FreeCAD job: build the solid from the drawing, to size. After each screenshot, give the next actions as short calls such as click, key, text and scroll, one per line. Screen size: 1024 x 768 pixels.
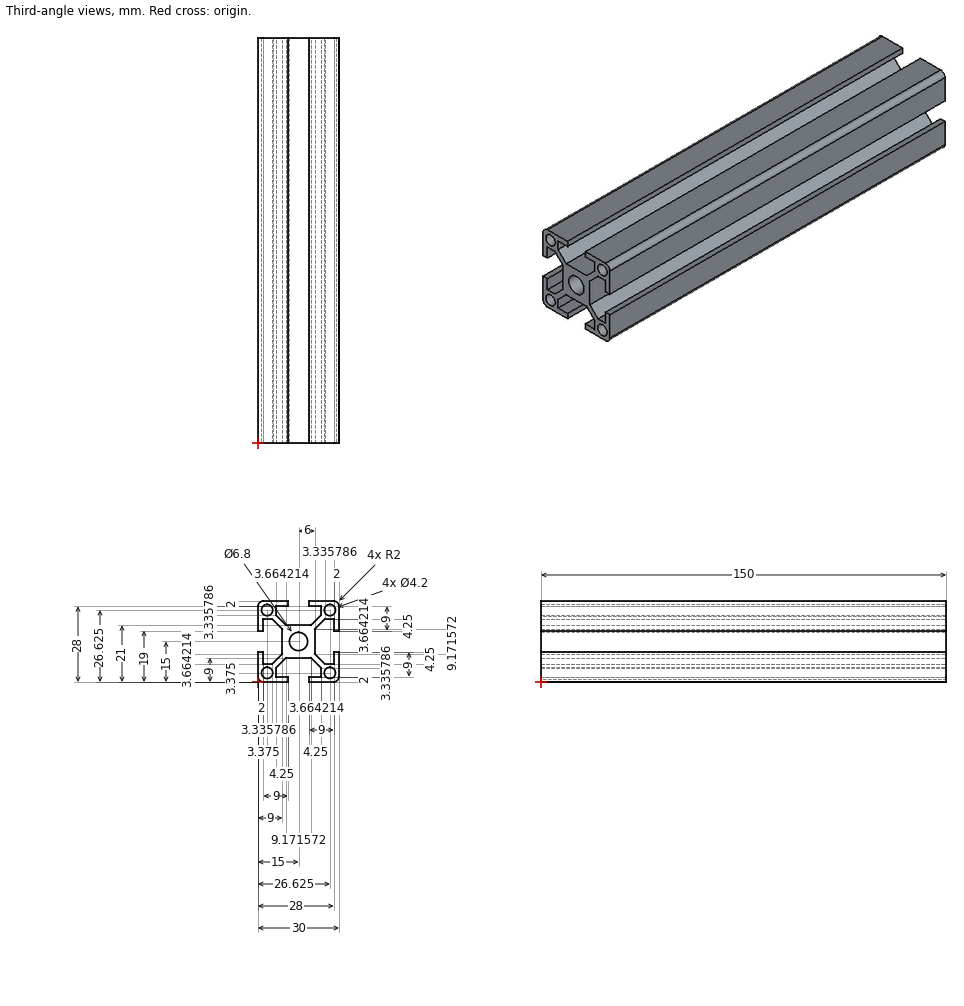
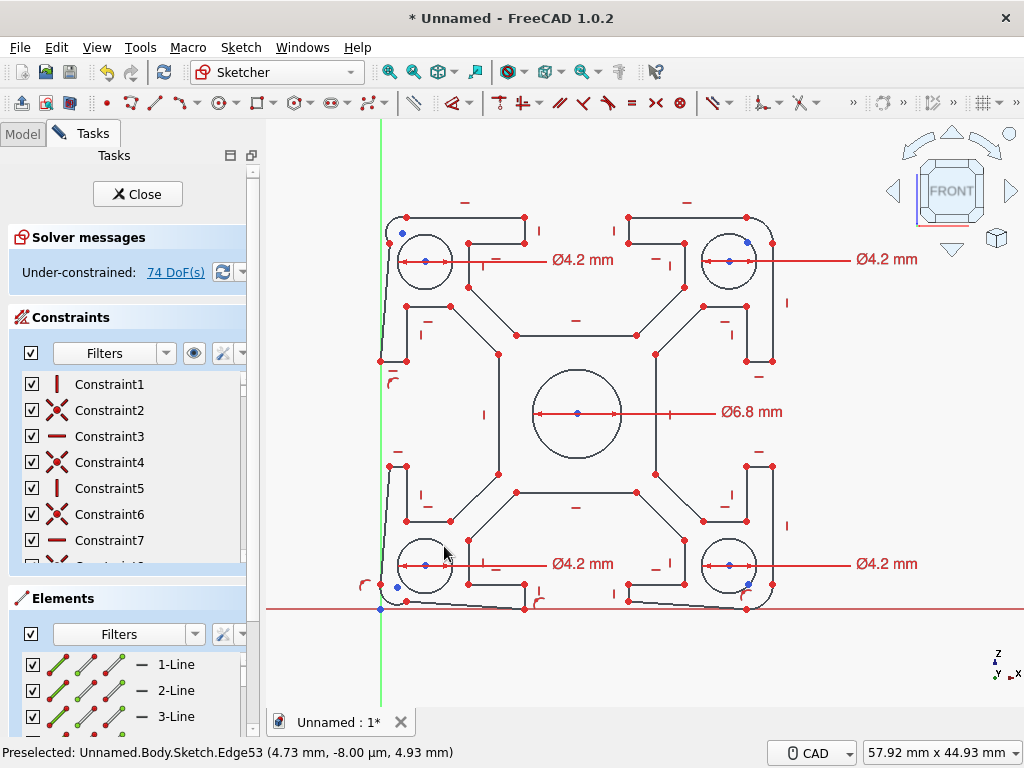
click(773, 279)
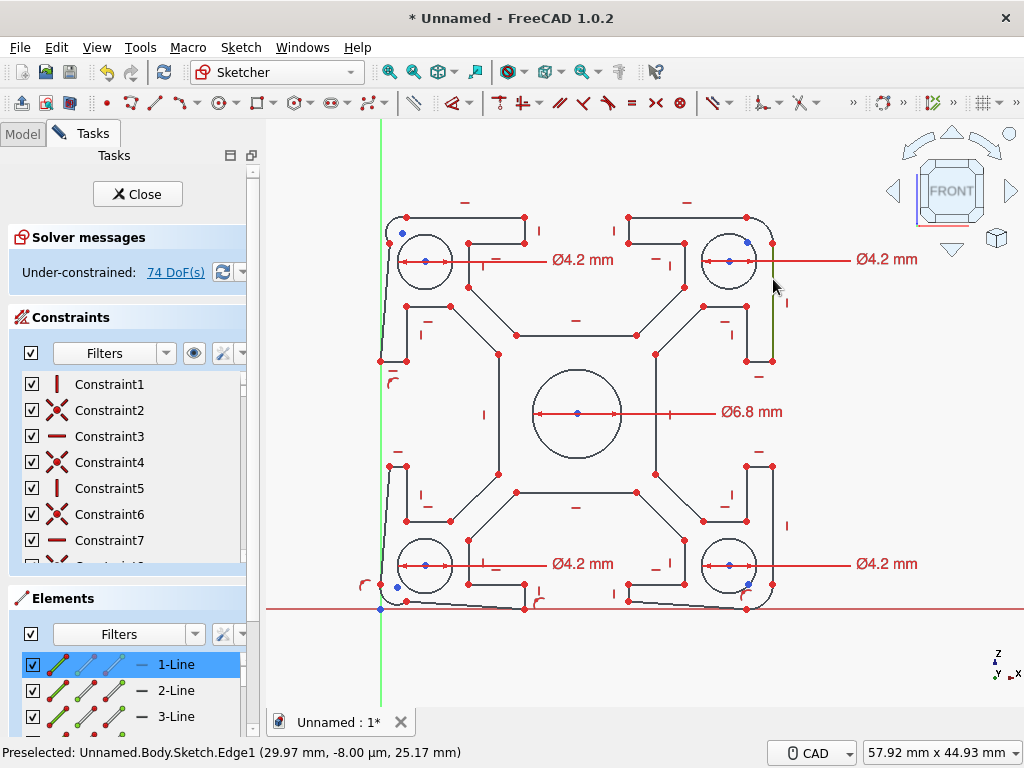
click(770, 232)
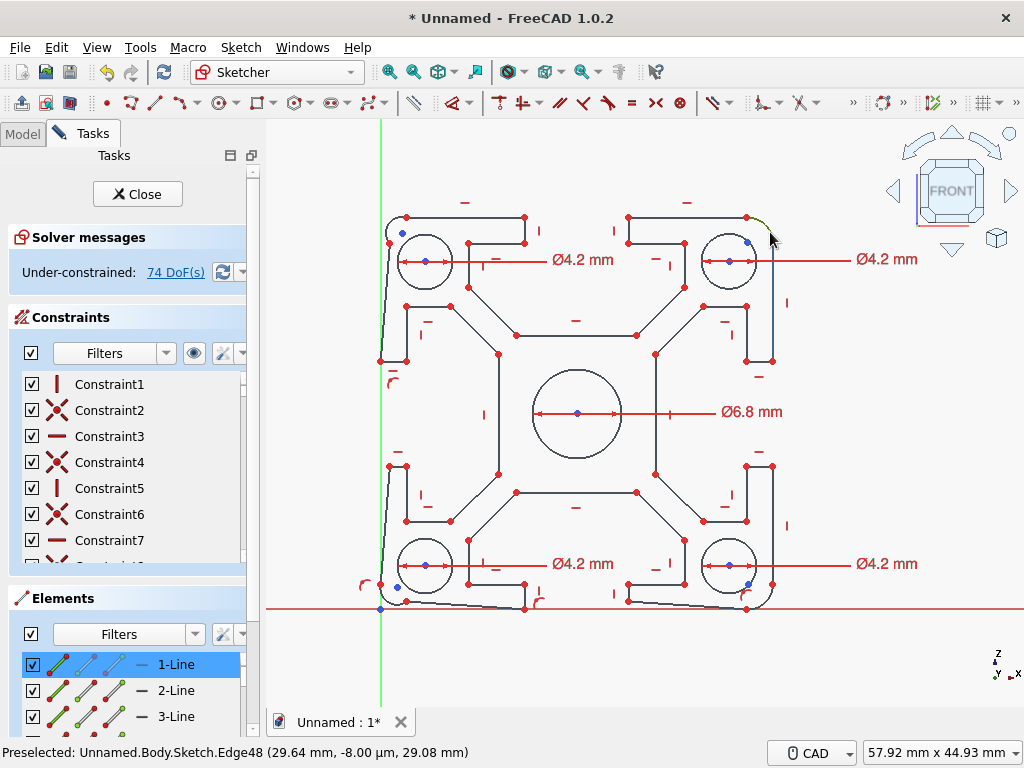
click(608, 104)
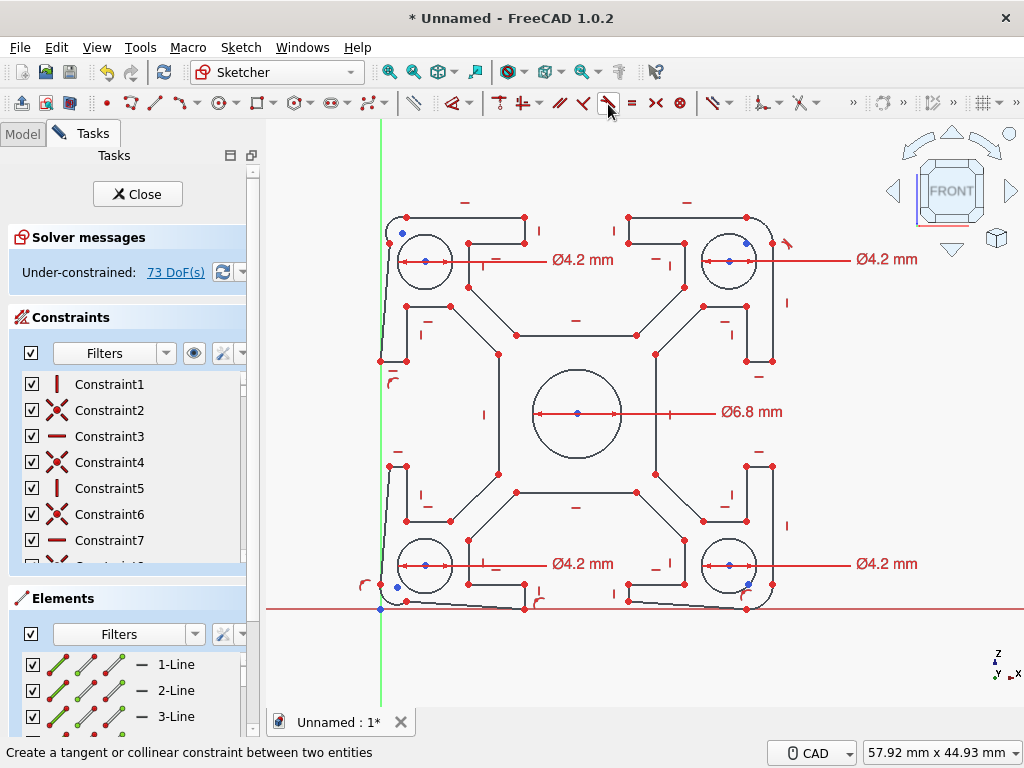
click(773, 502)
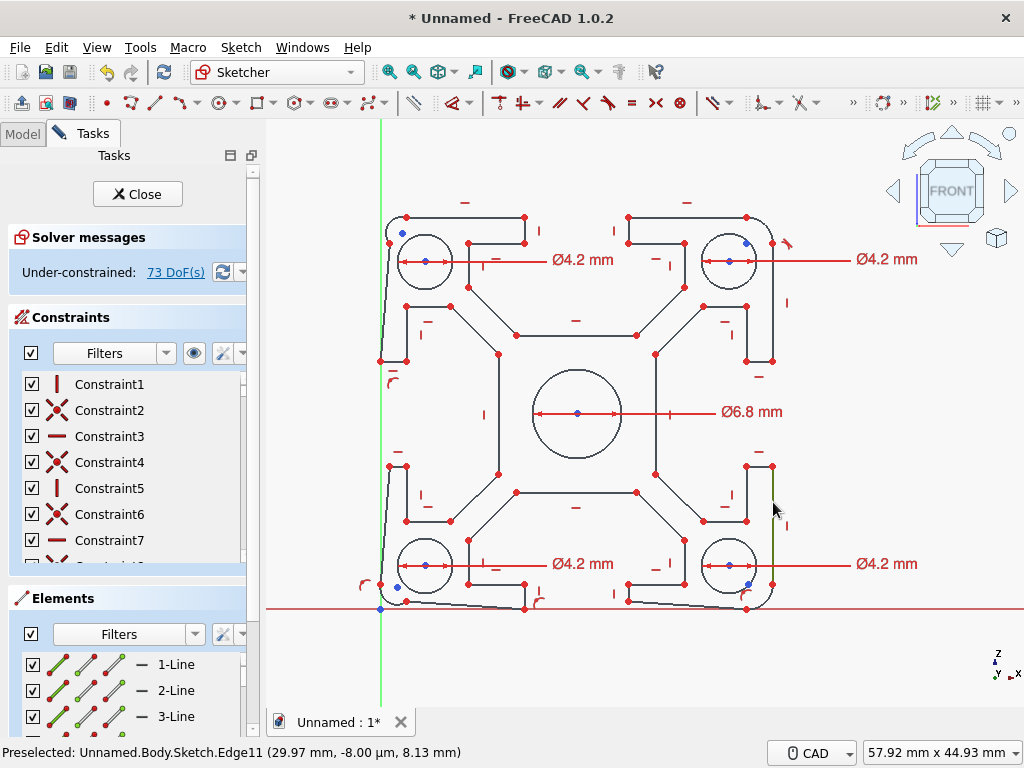
click(759, 607)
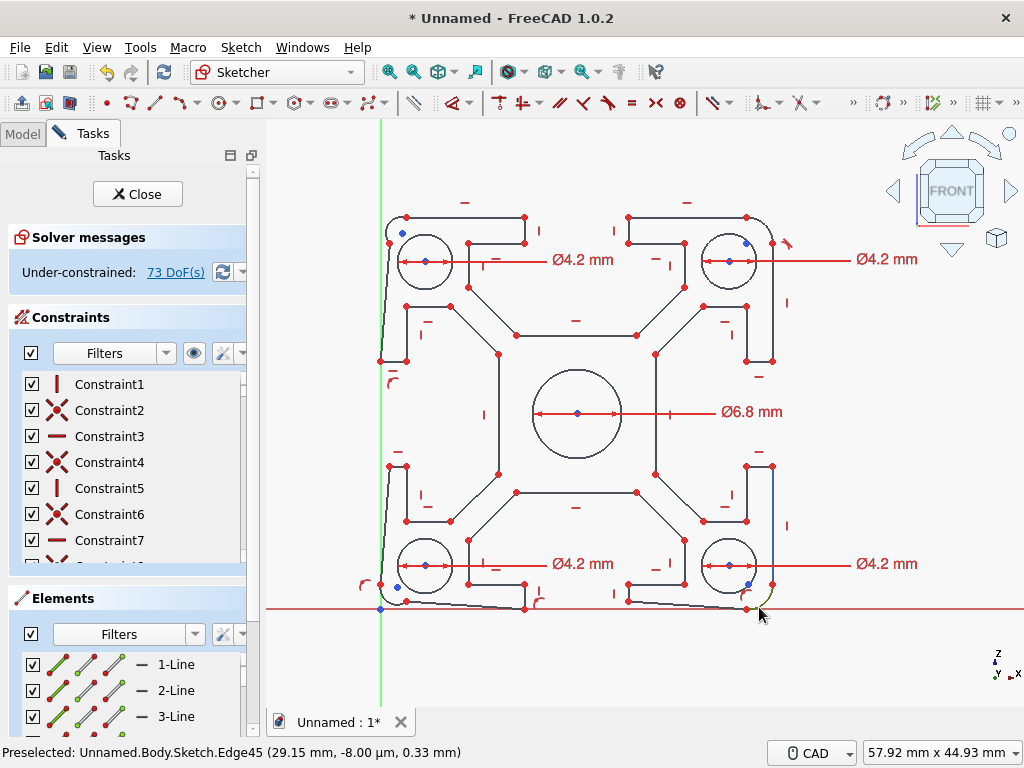
key(t)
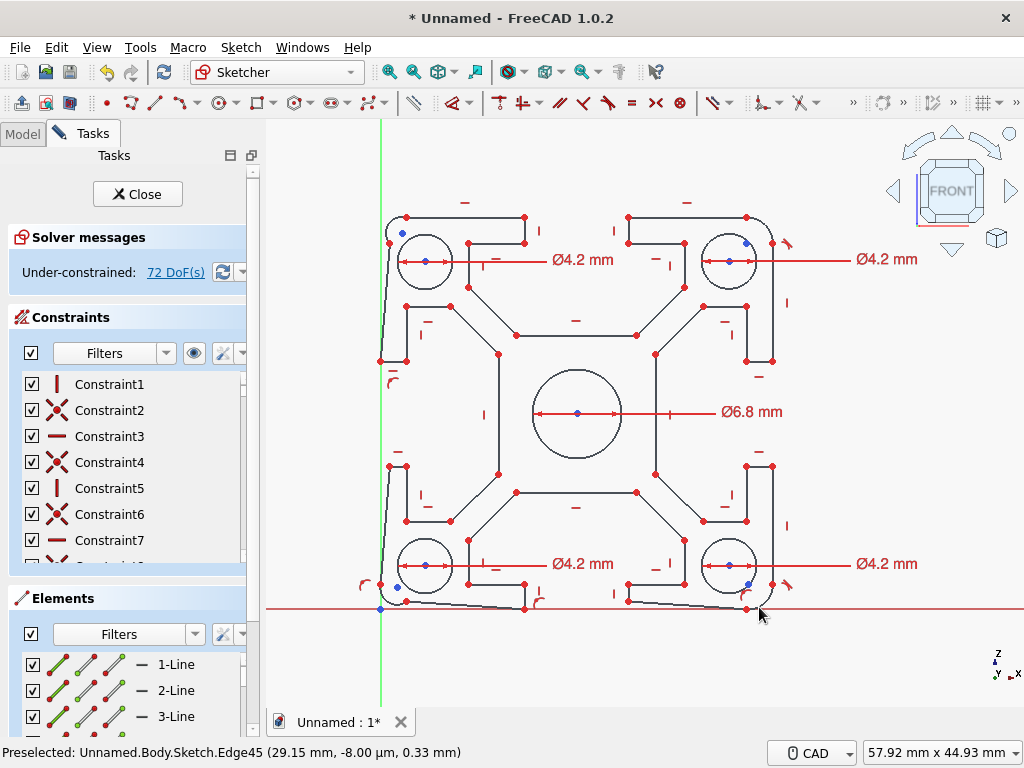
click(711, 607)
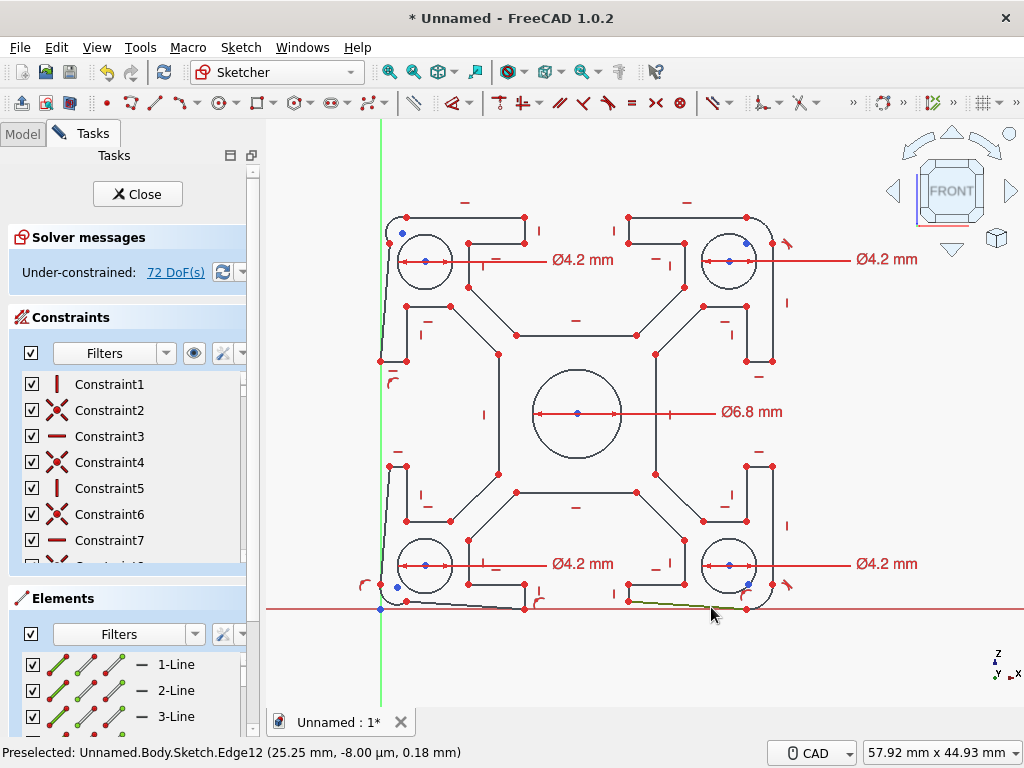
click(759, 607)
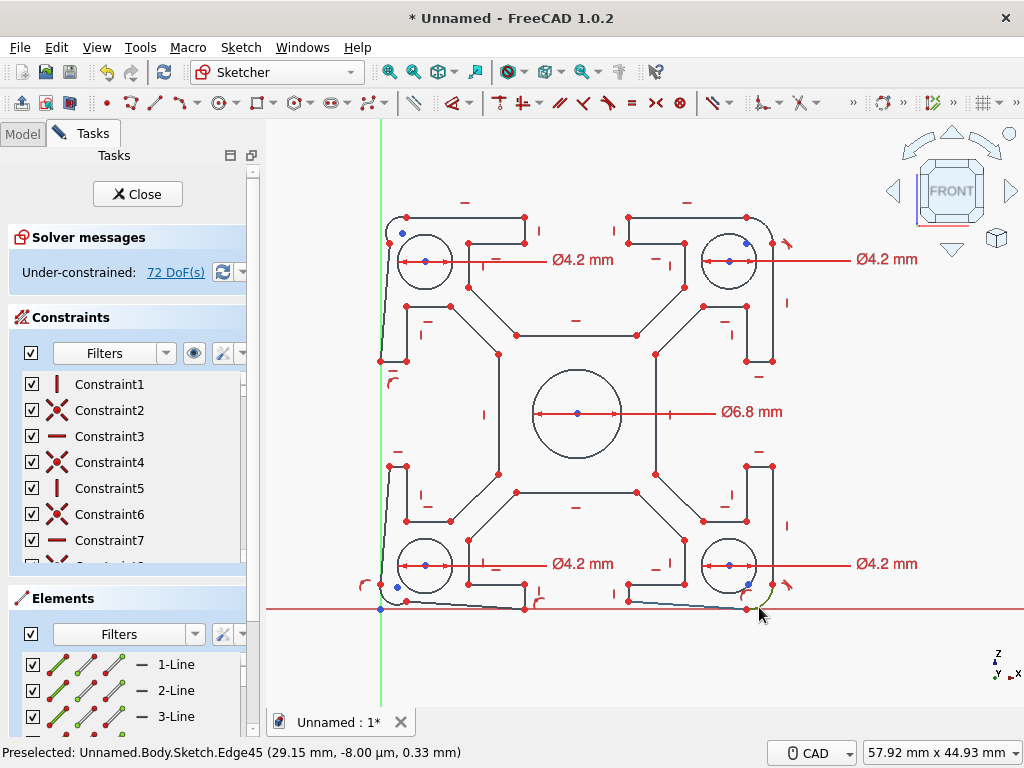
click(608, 104)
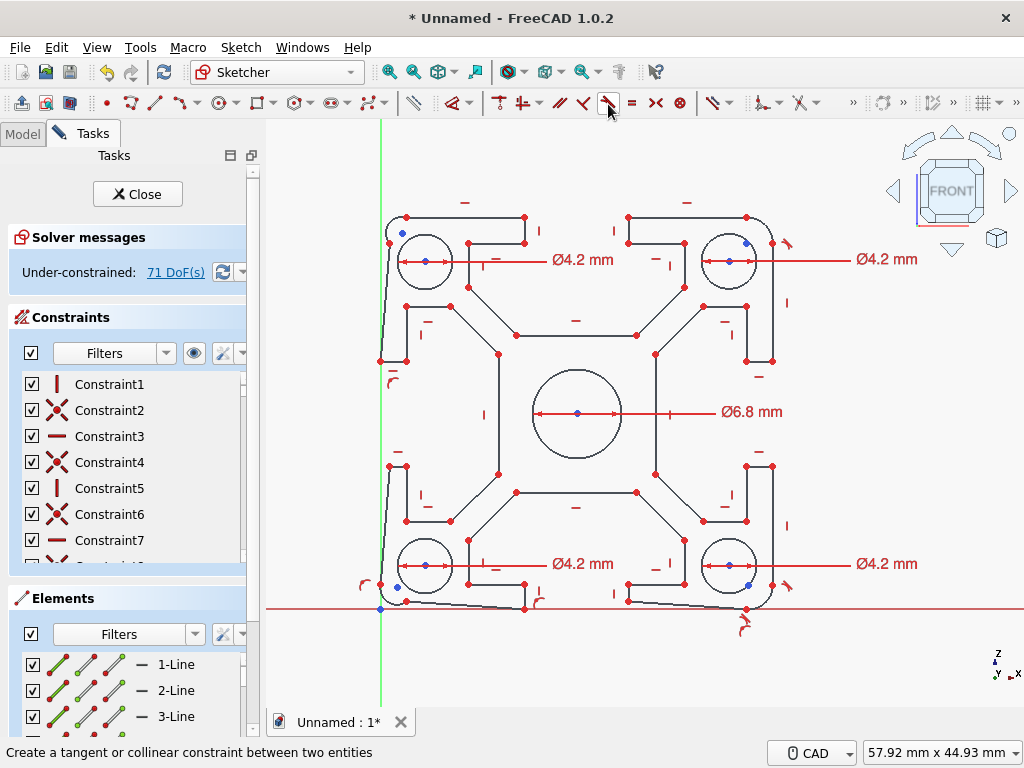
click(489, 607)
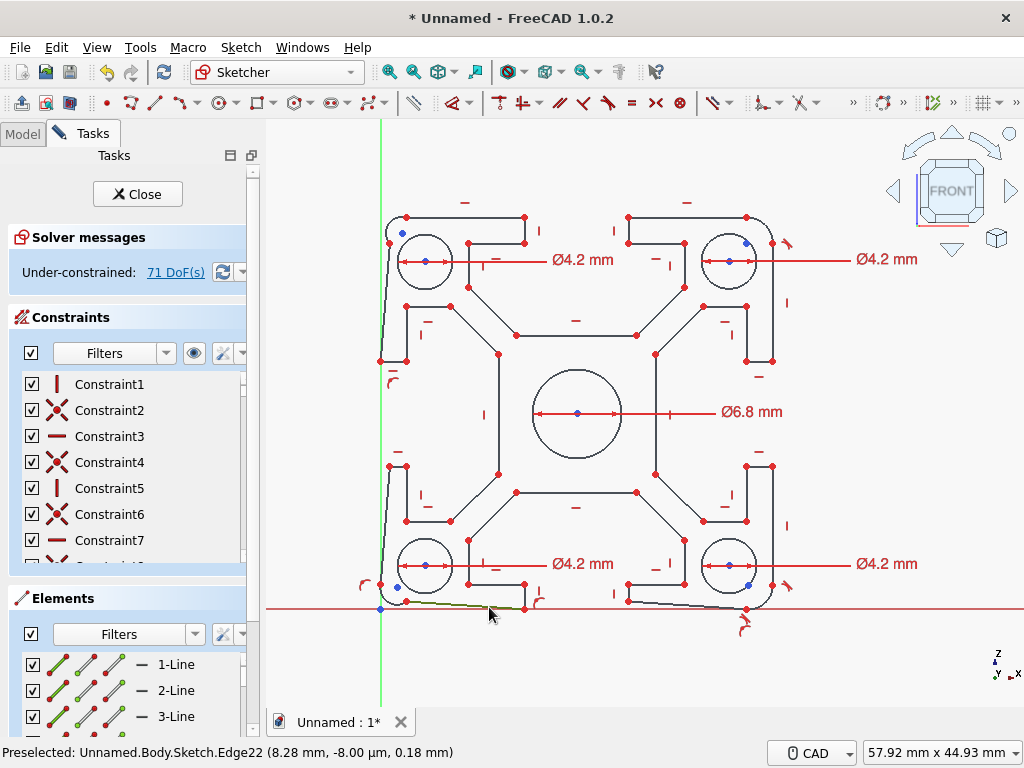
click(383, 596)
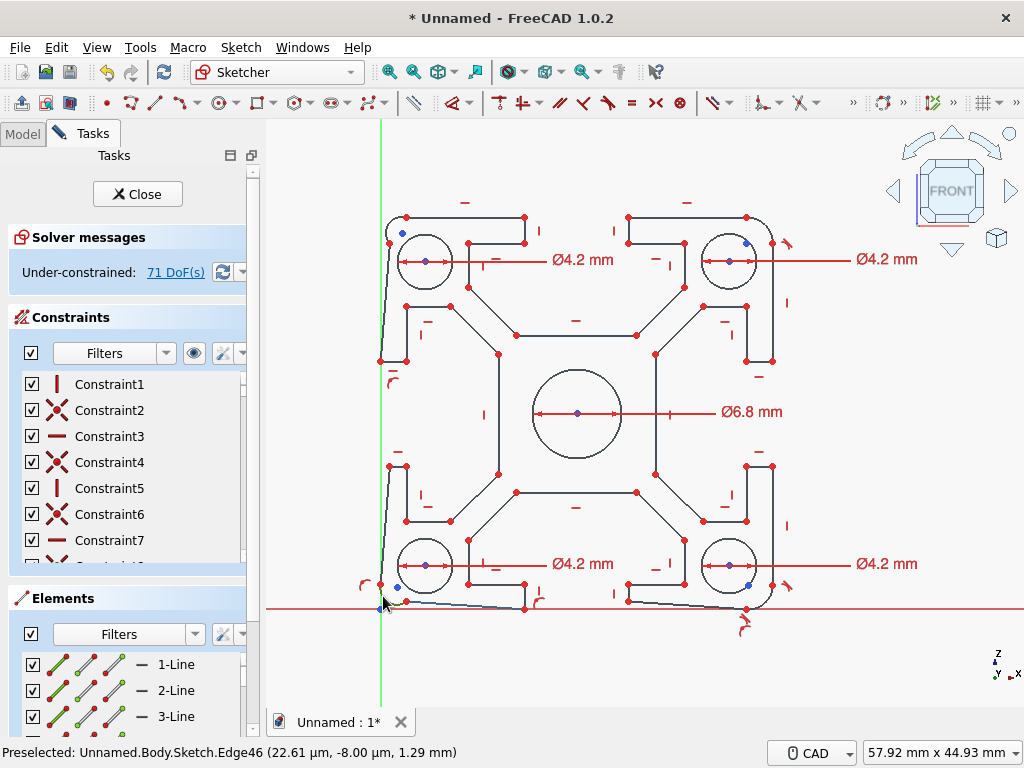
key(t)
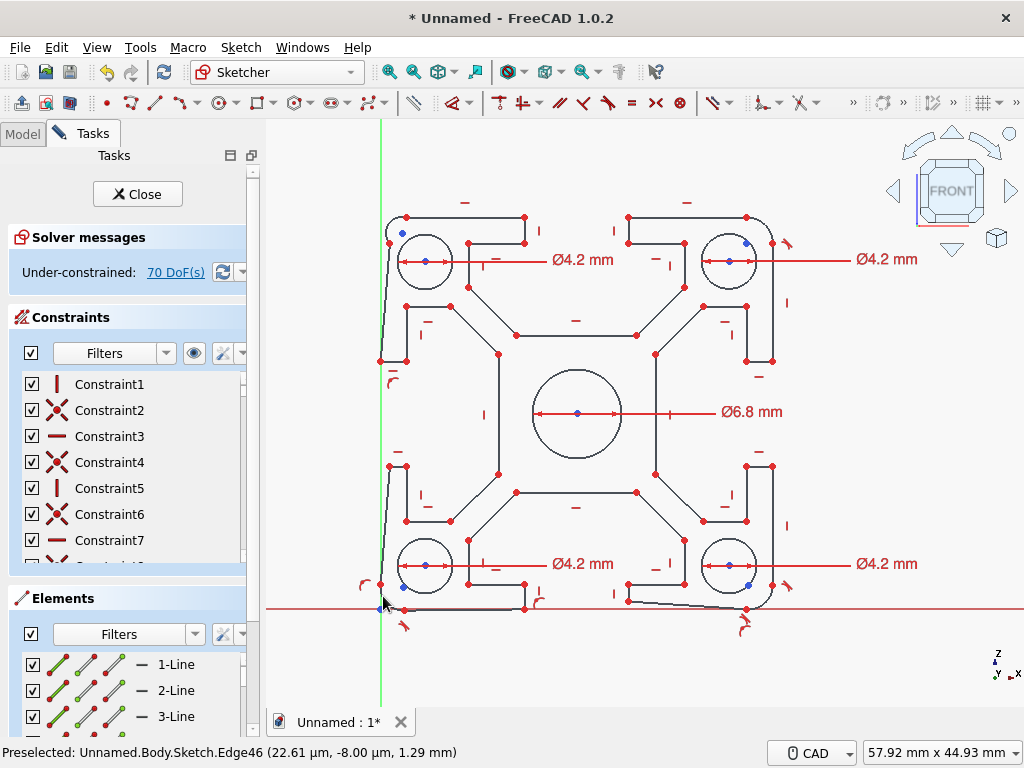
click(383, 549)